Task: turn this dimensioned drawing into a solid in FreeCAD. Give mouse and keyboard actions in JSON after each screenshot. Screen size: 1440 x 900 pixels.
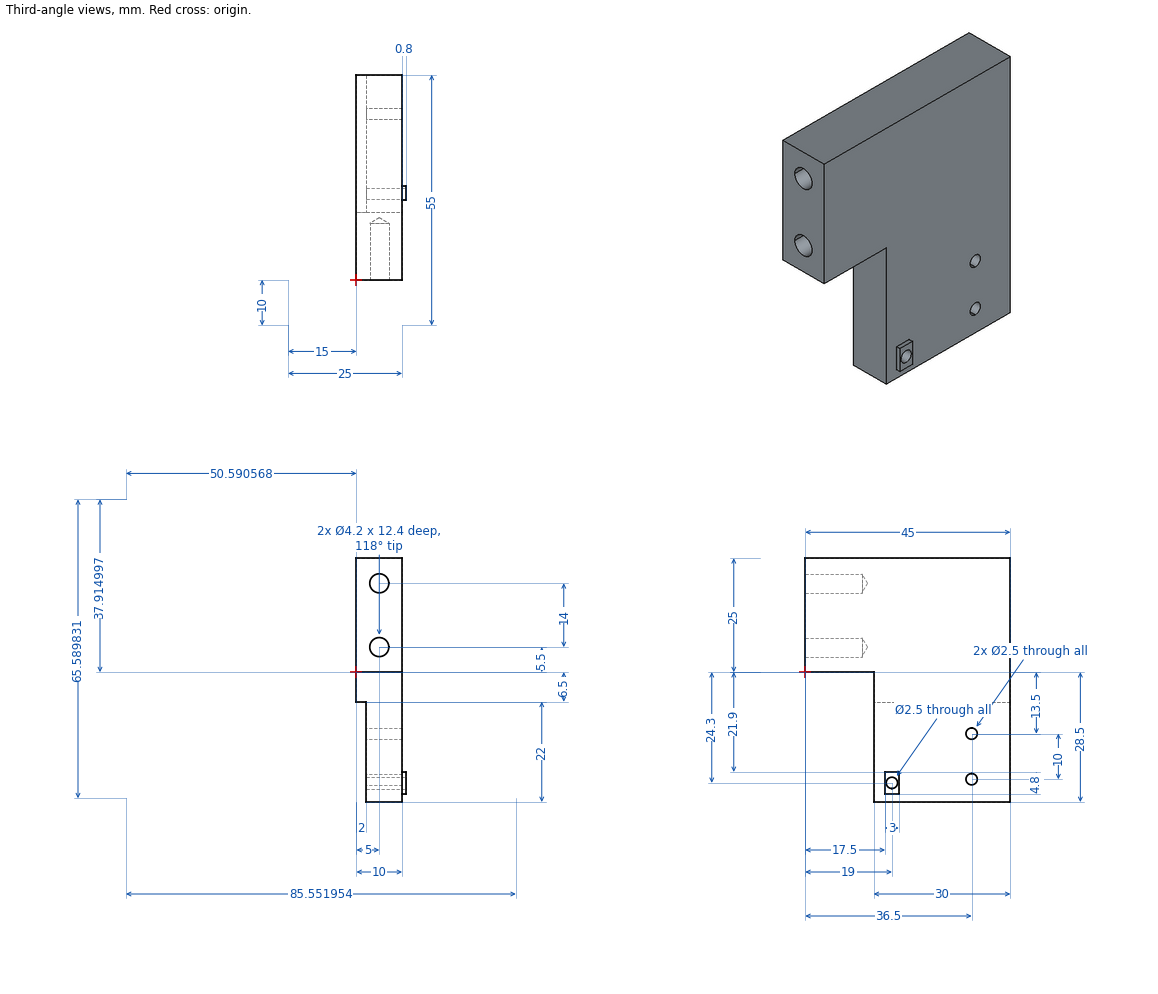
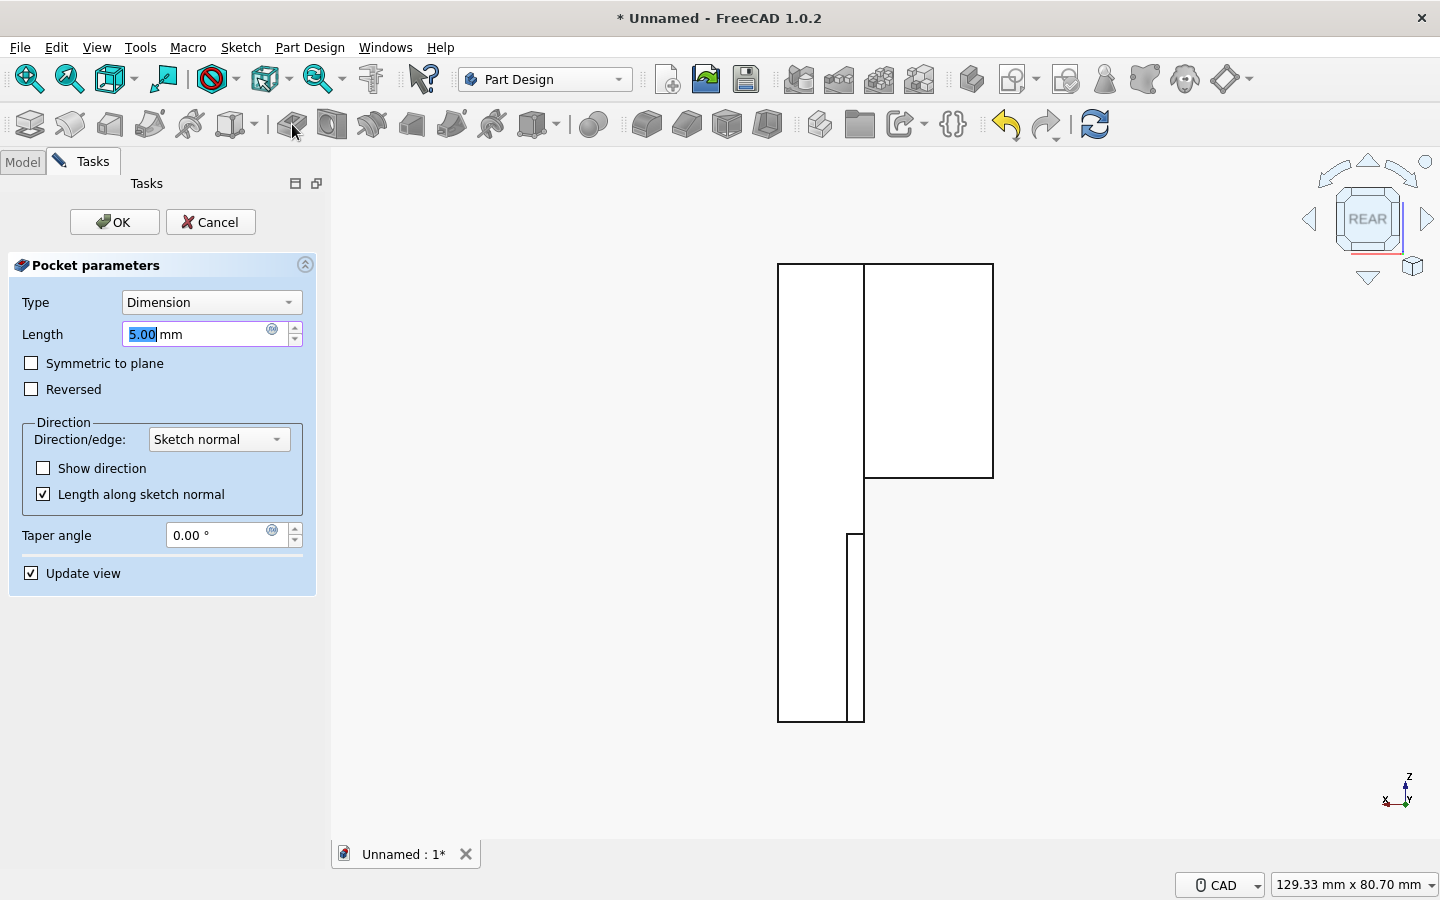
{"action": "left_click", "coordinate": [212, 302]}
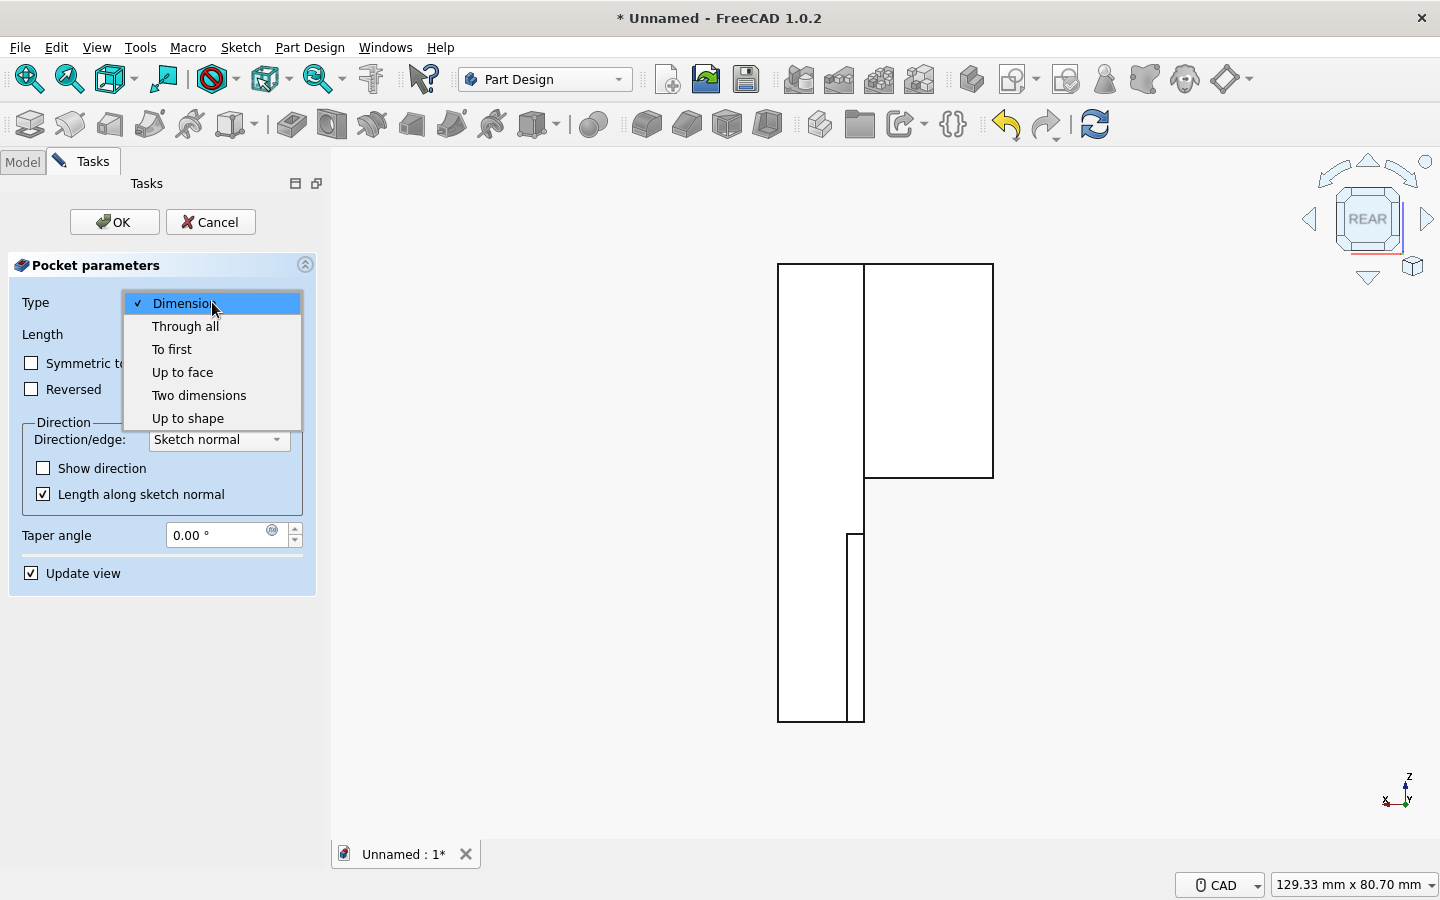
{"action": "left_click", "coordinate": [212, 326]}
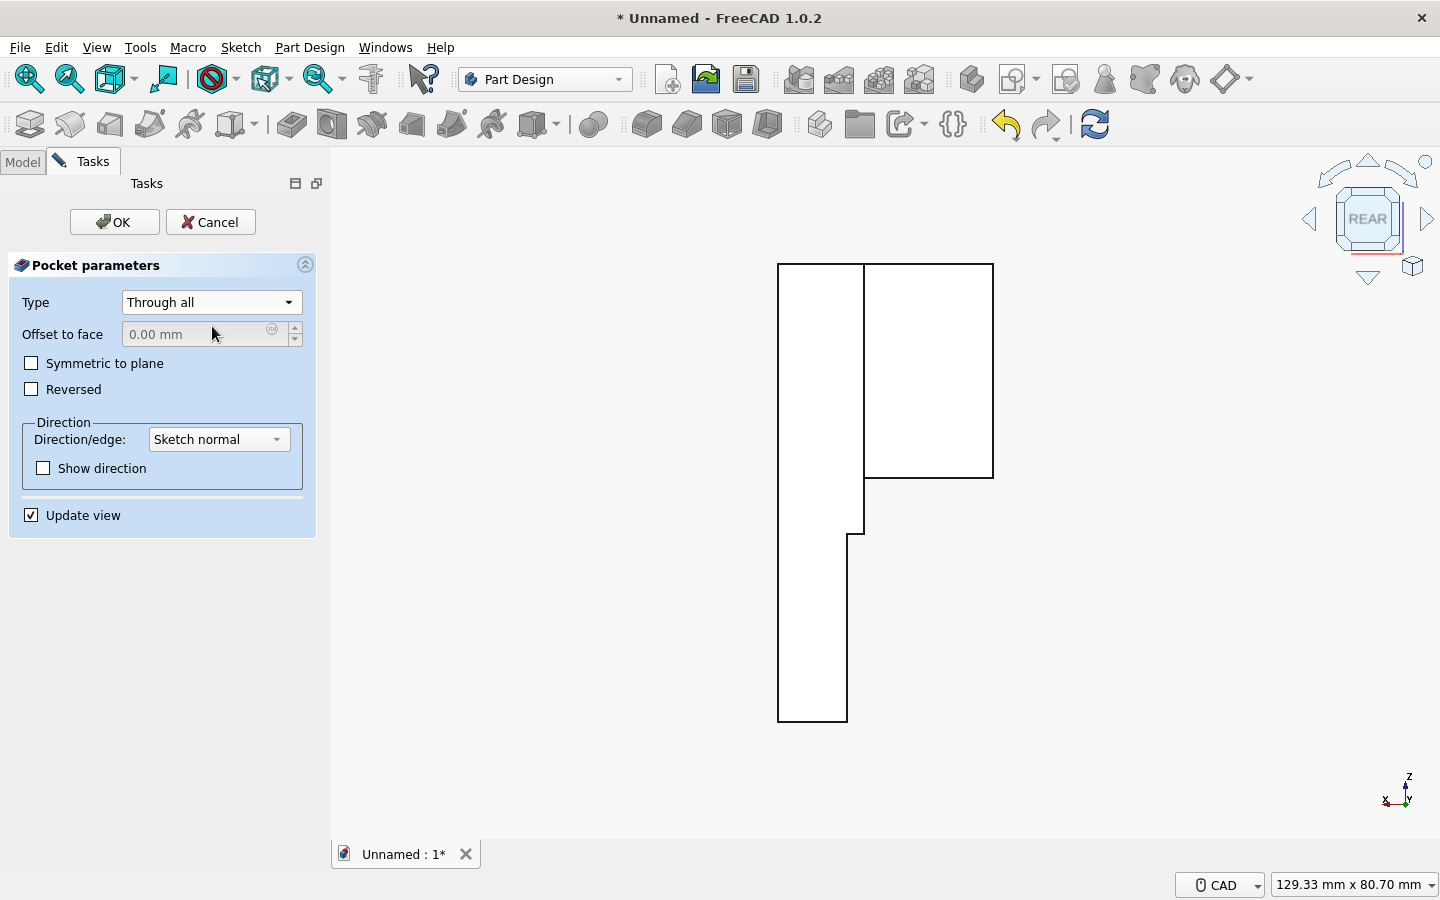
{"action": "left_click", "coordinate": [115, 222]}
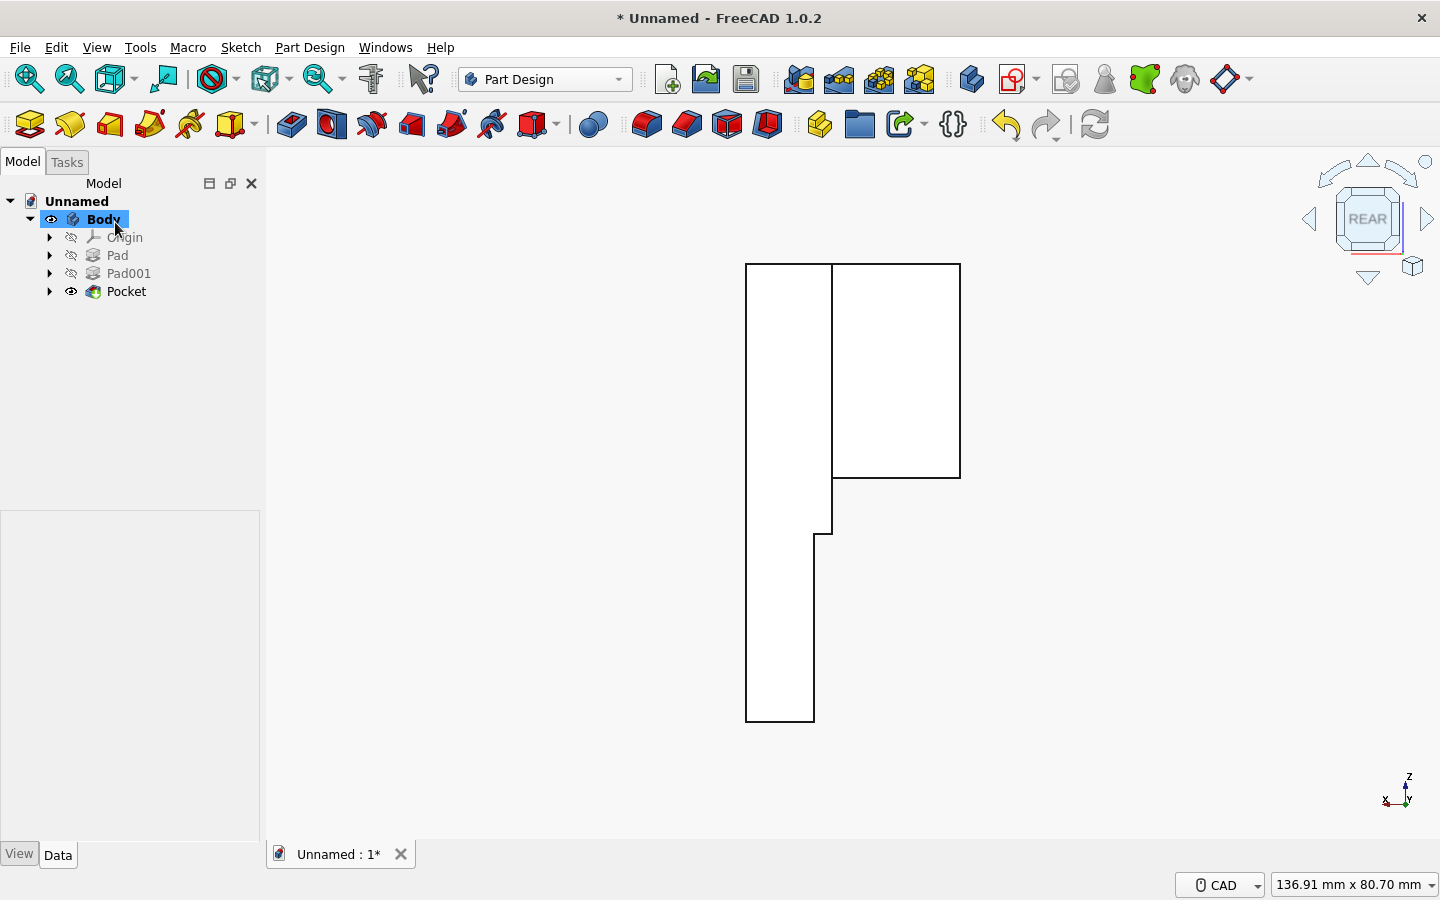
{"action": "key", "text": "0"}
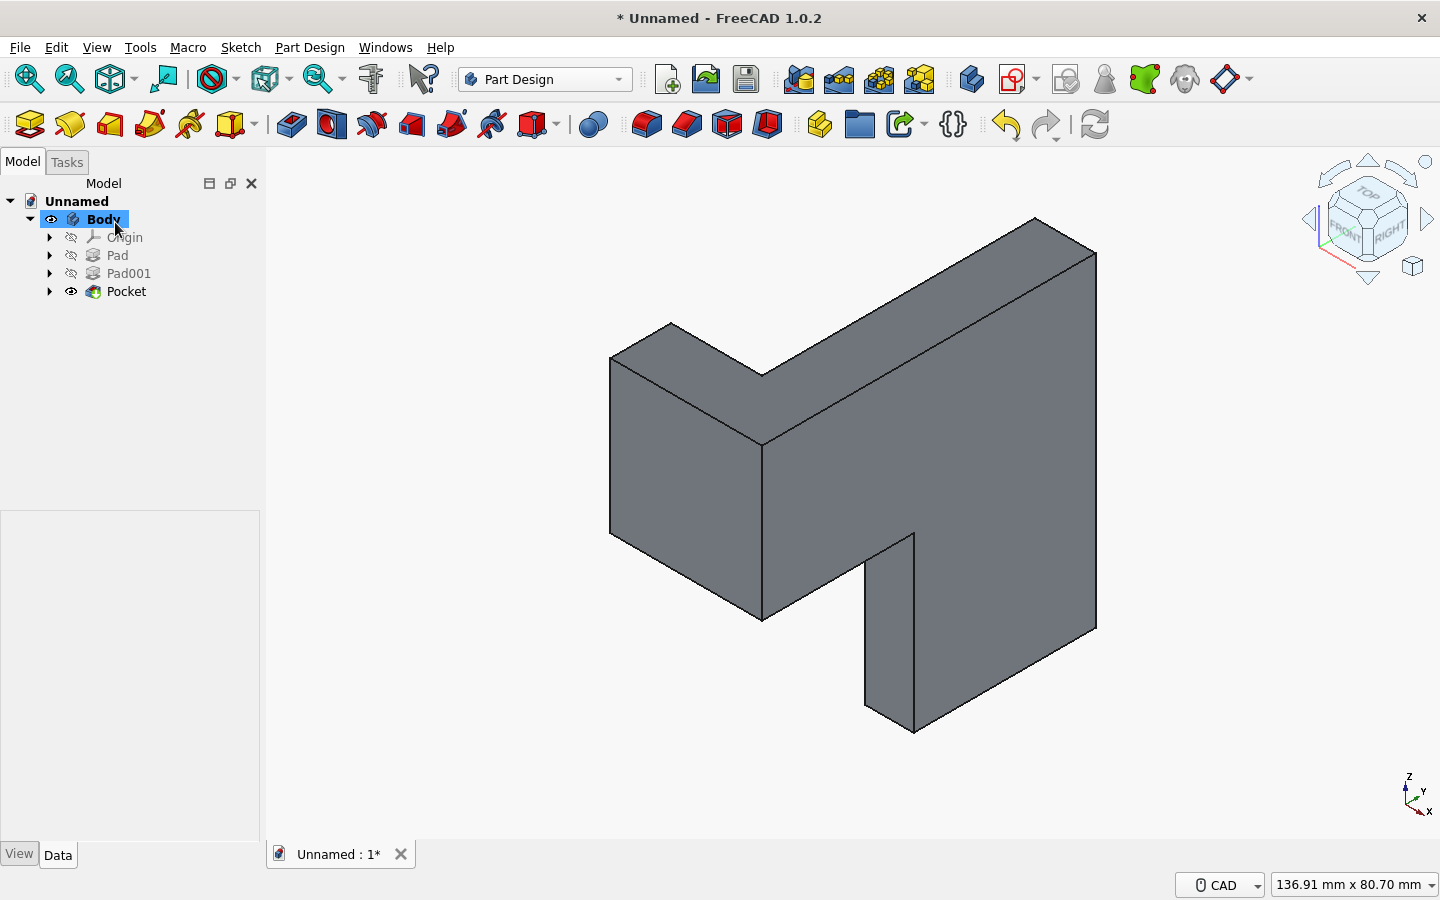
{"action": "left_click", "coordinate": [976, 455]}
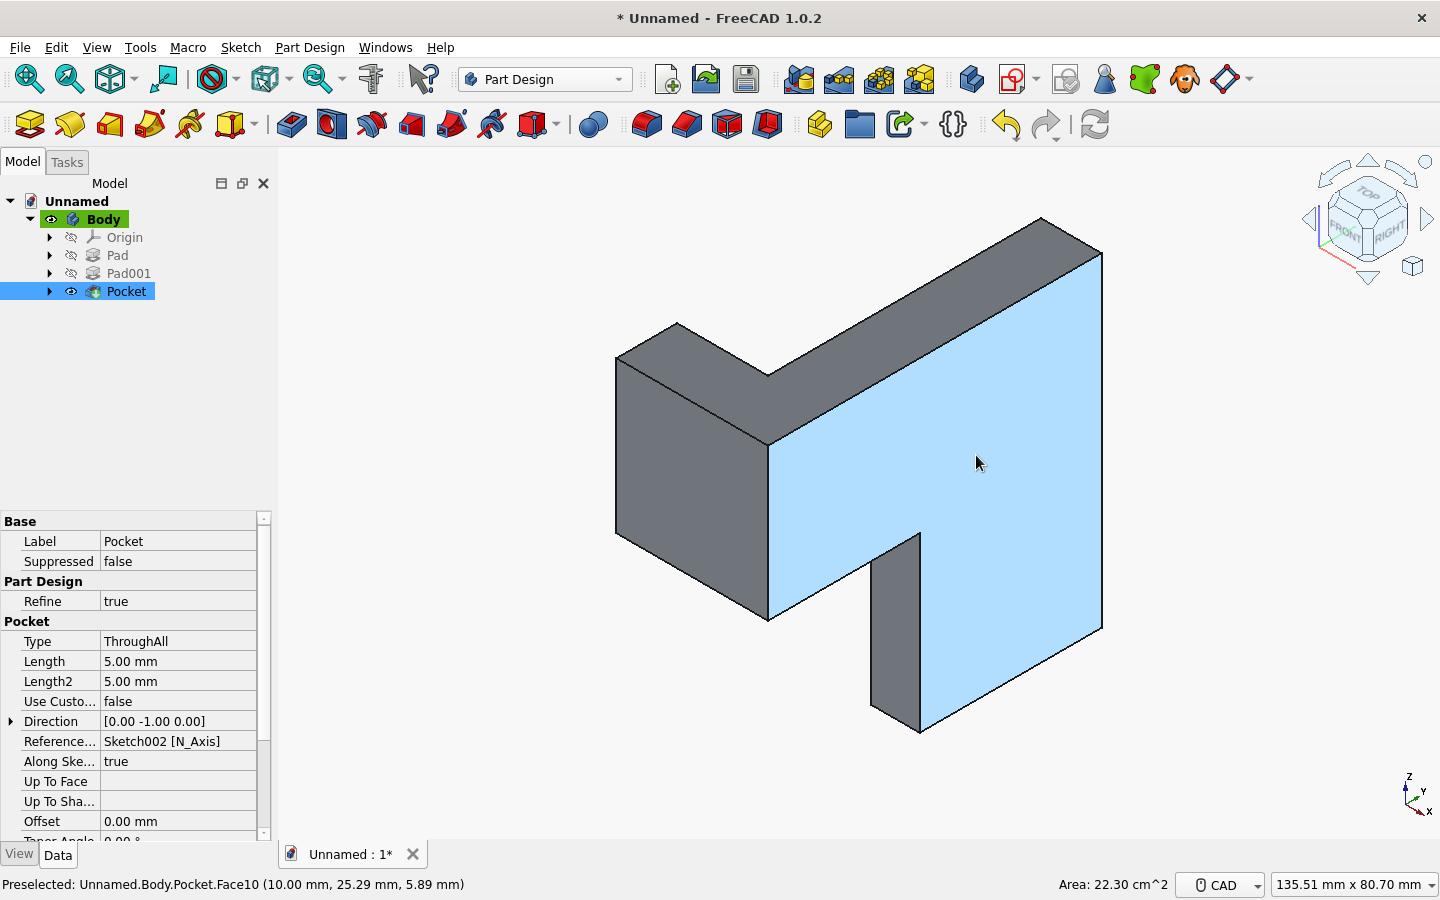
{"action": "left_click", "coordinate": [1012, 80]}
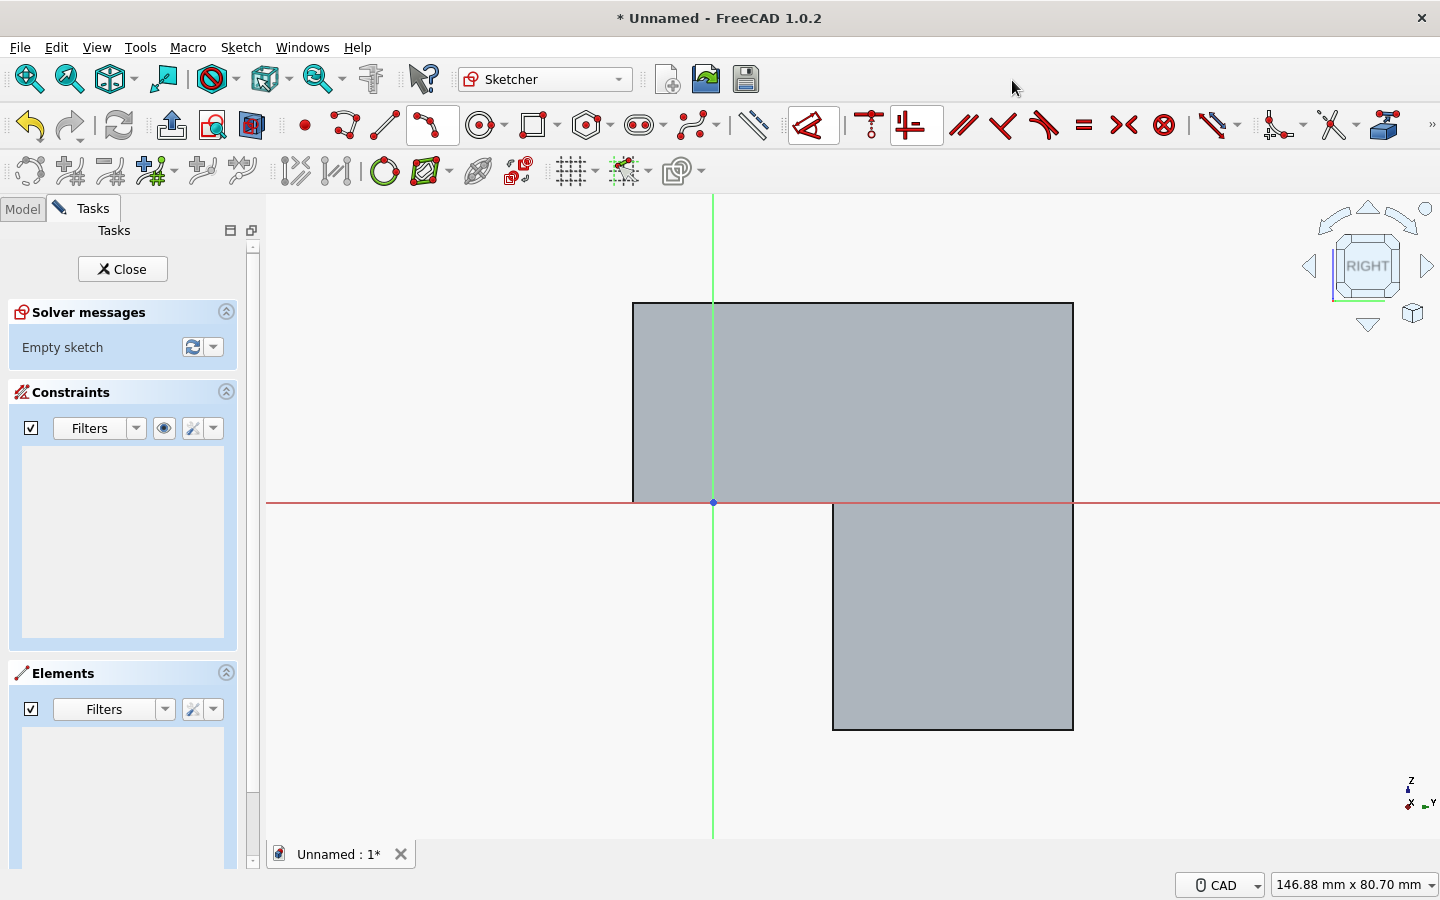
{"action": "scroll", "coordinate": [1077, 694], "scroll_direction": "up", "scroll_amount": 7}